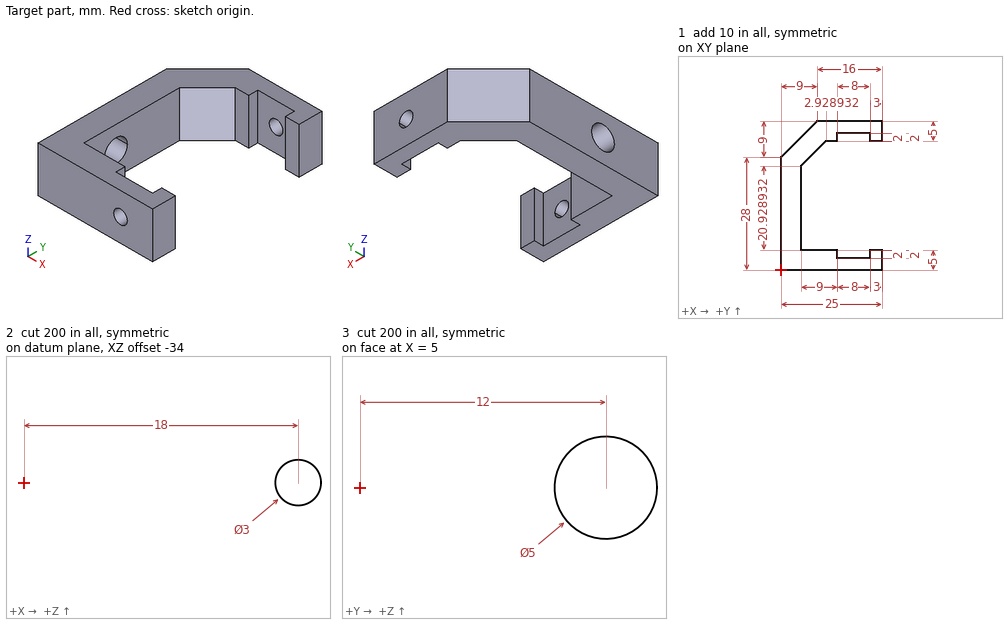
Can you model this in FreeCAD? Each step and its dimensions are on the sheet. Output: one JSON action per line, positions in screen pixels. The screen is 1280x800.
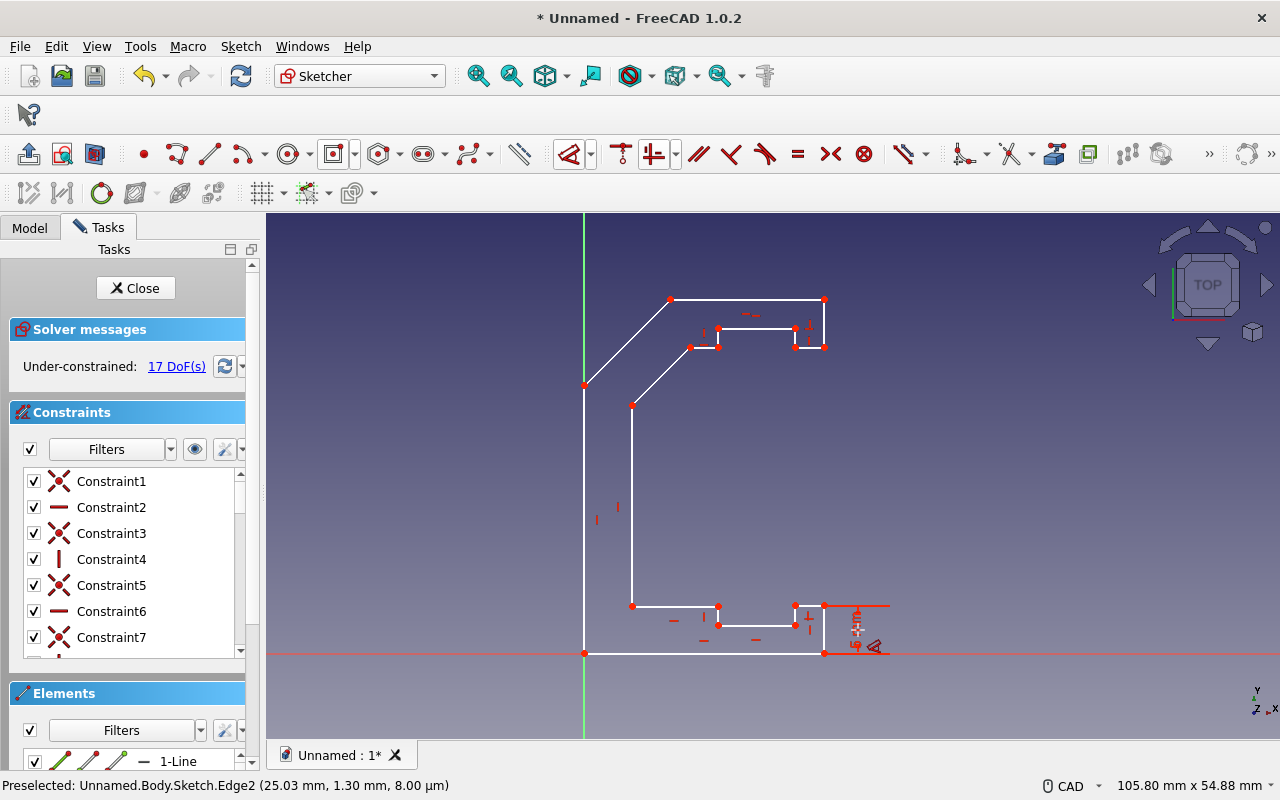
{"action": "scroll", "coordinate": [812, 606], "scroll_direction": "up", "scroll_amount": 2}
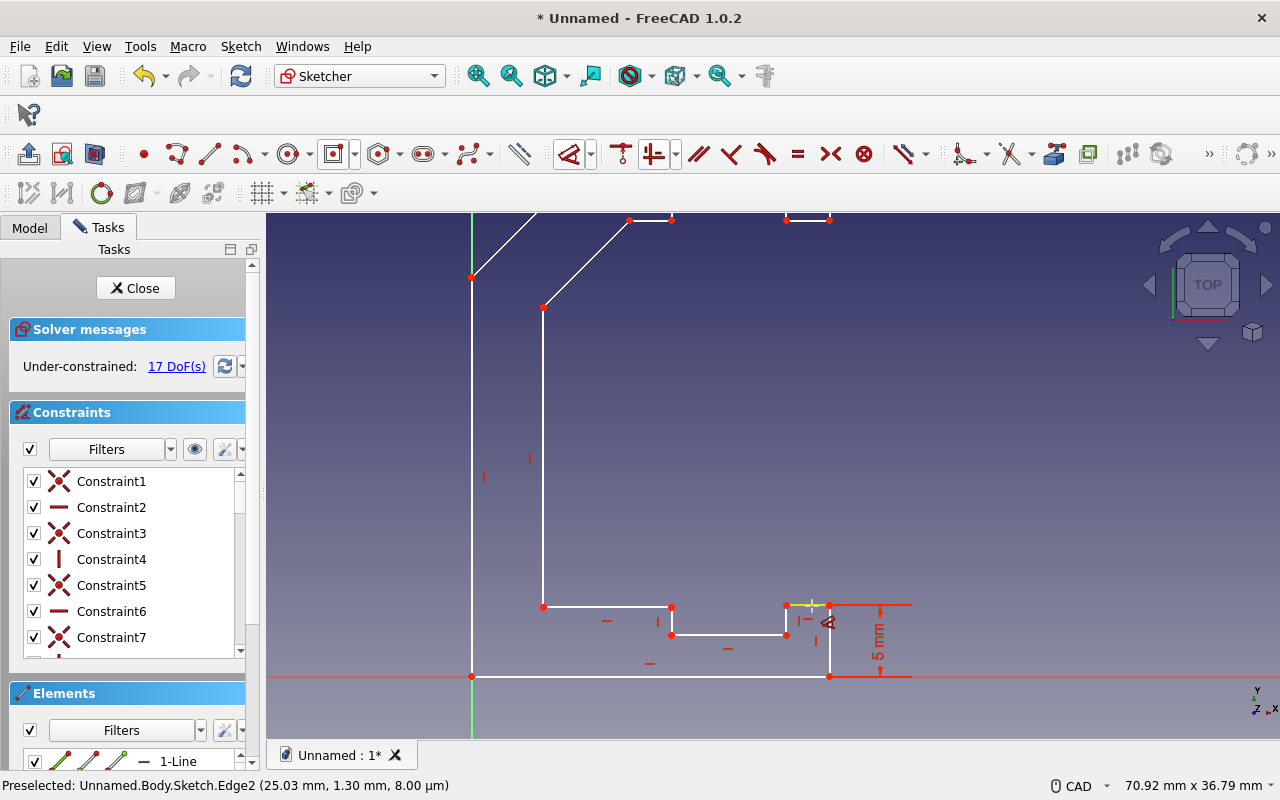
{"action": "left_click", "coordinate": [812, 605]}
{"action": "left_click", "coordinate": [808, 639]}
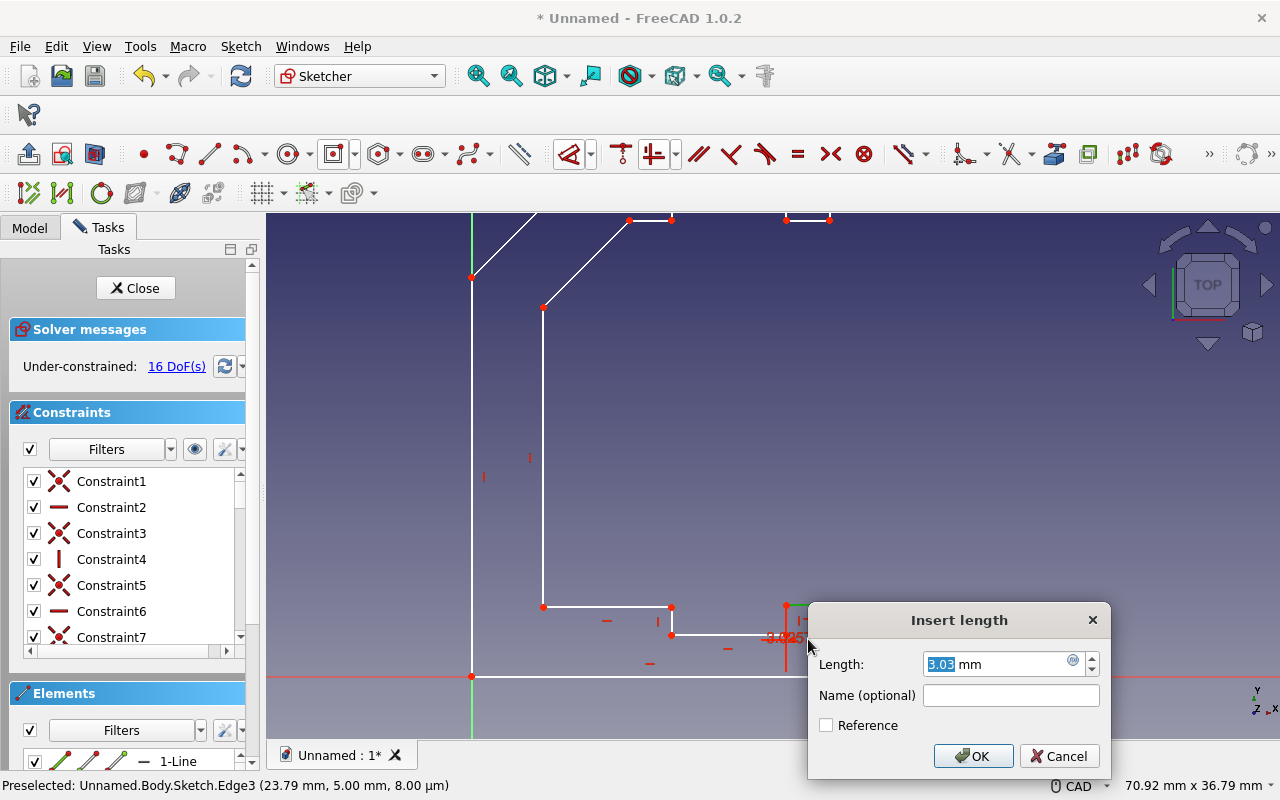
{"action": "type", "text": "3"}
{"action": "key", "text": "Return"}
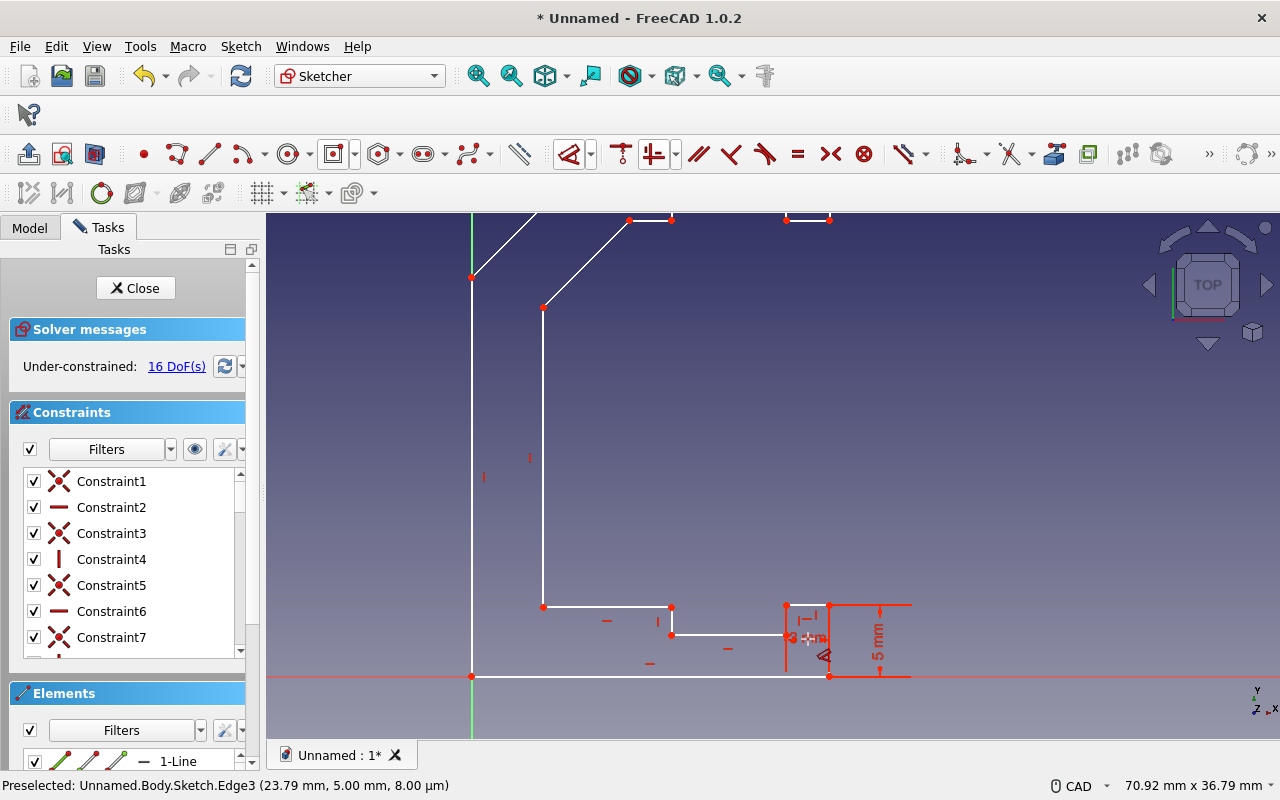
{"action": "scroll", "coordinate": [786, 614], "scroll_direction": "up", "scroll_amount": 3}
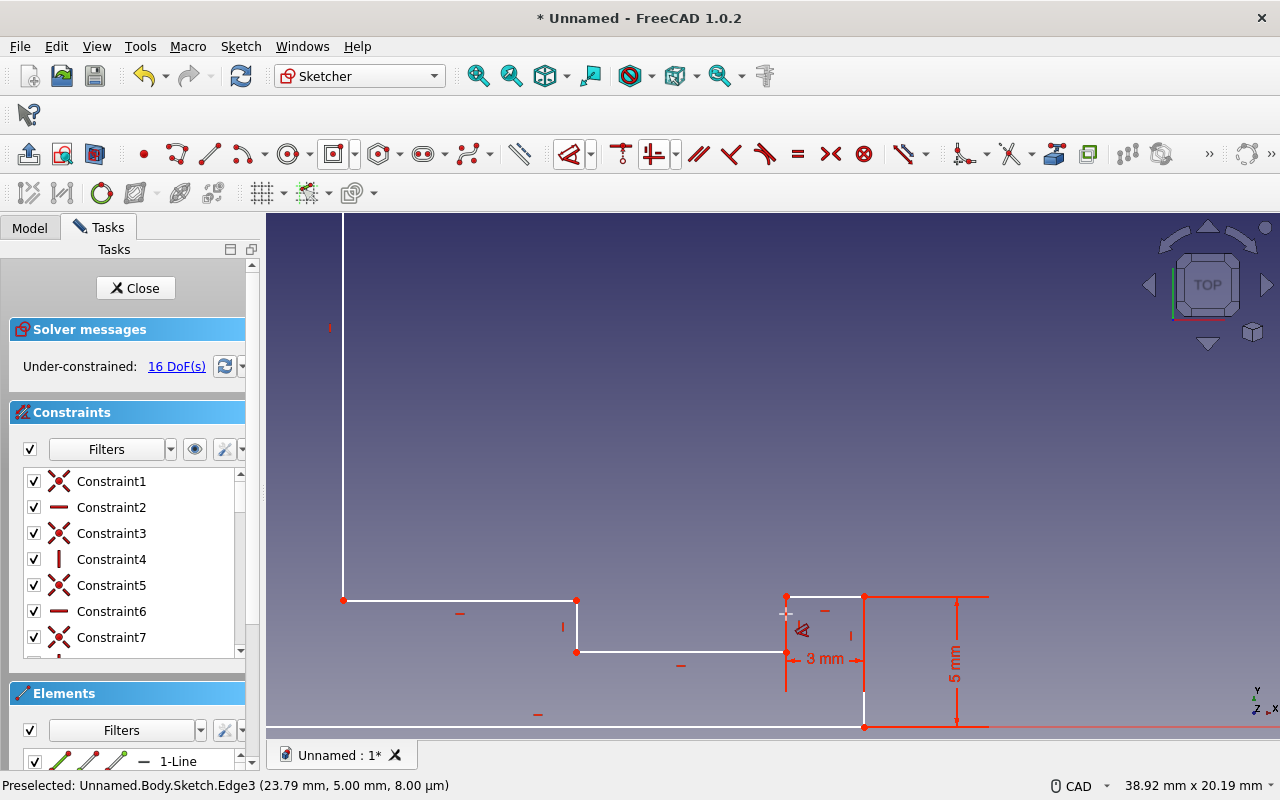
{"action": "left_click", "coordinate": [786, 614]}
{"action": "left_click", "coordinate": [820, 625]}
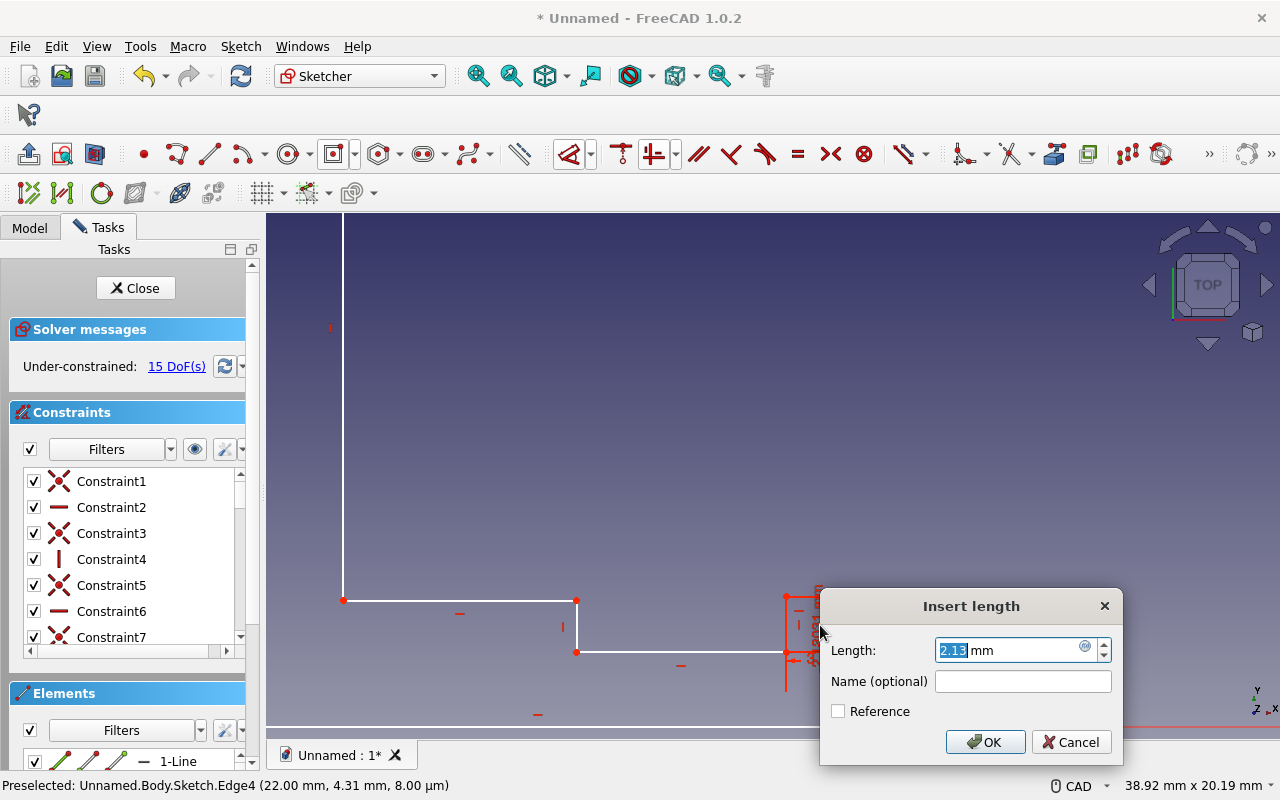
{"action": "type", "text": "2"}
{"action": "key", "text": "Return"}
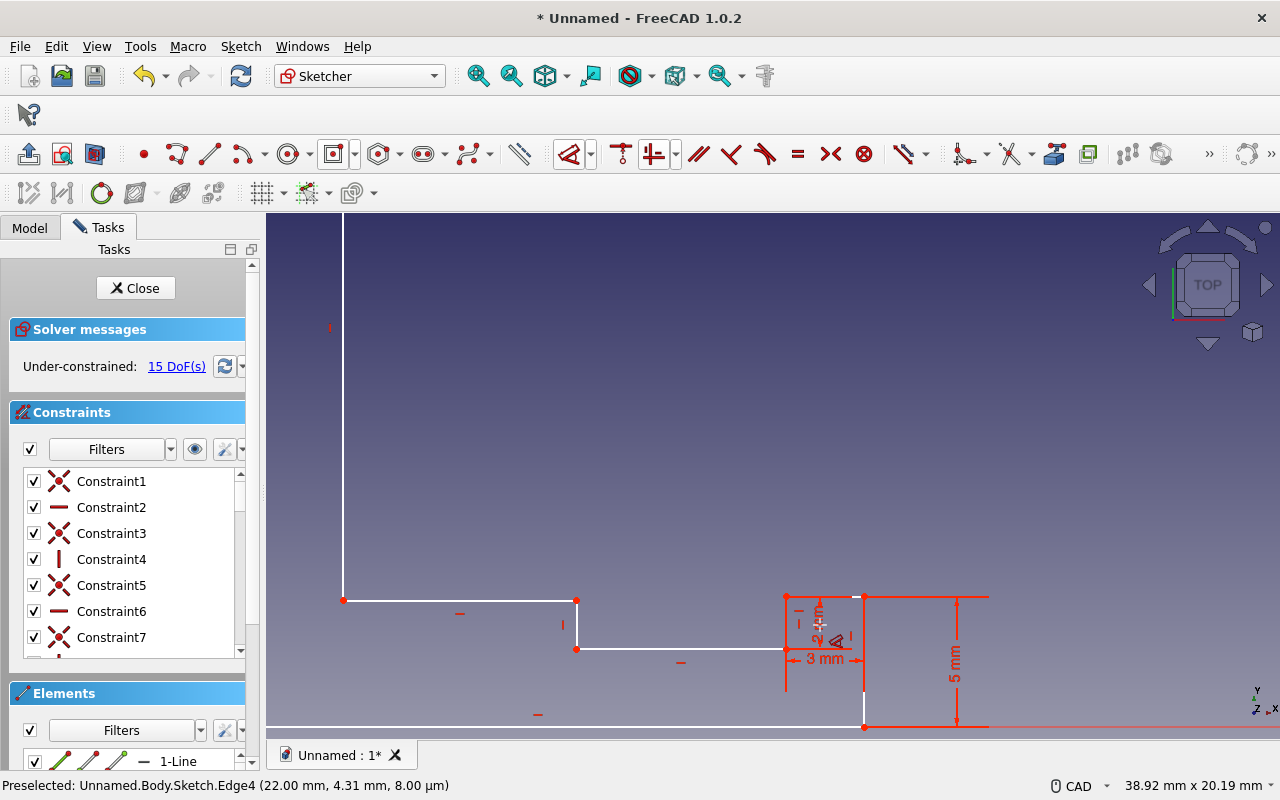
{"action": "left_click", "coordinate": [723, 649]}
{"action": "left_click", "coordinate": [682, 683]}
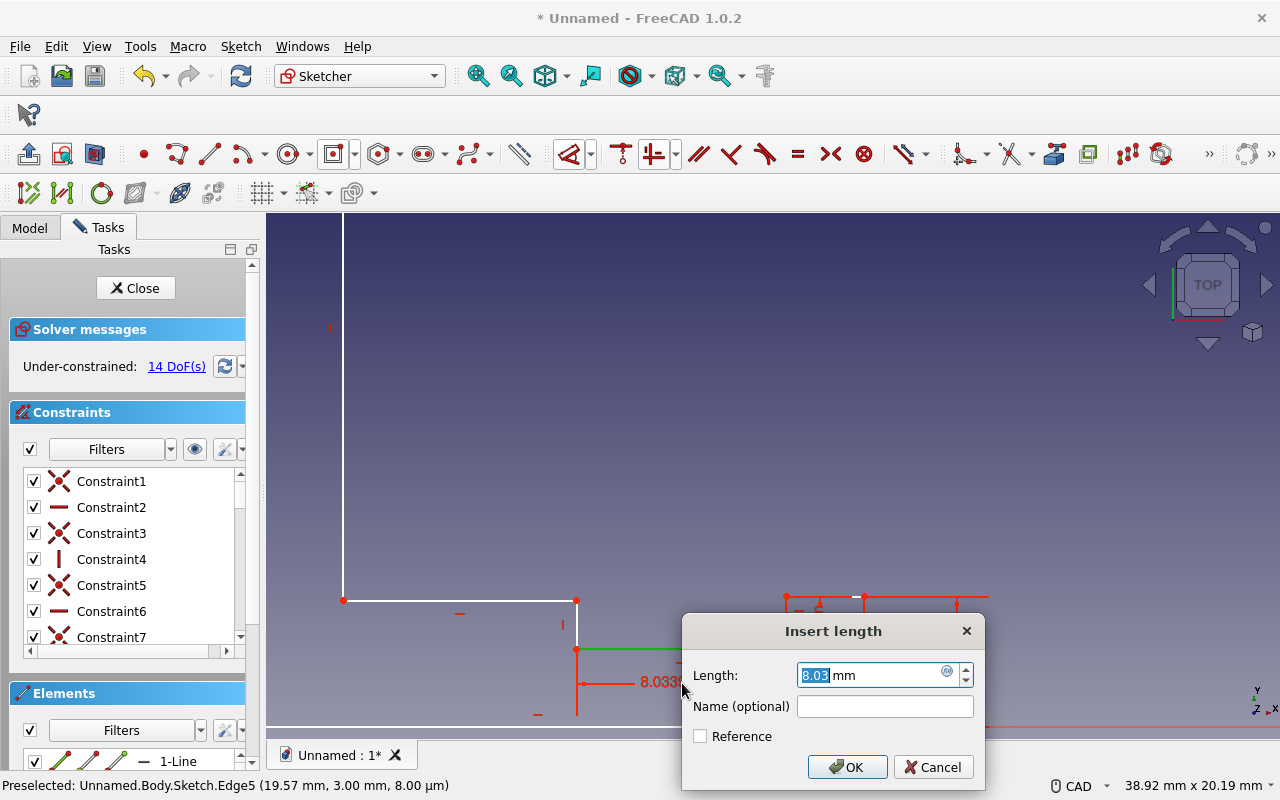
{"action": "type", "text": "8"}
{"action": "key", "text": "Return"}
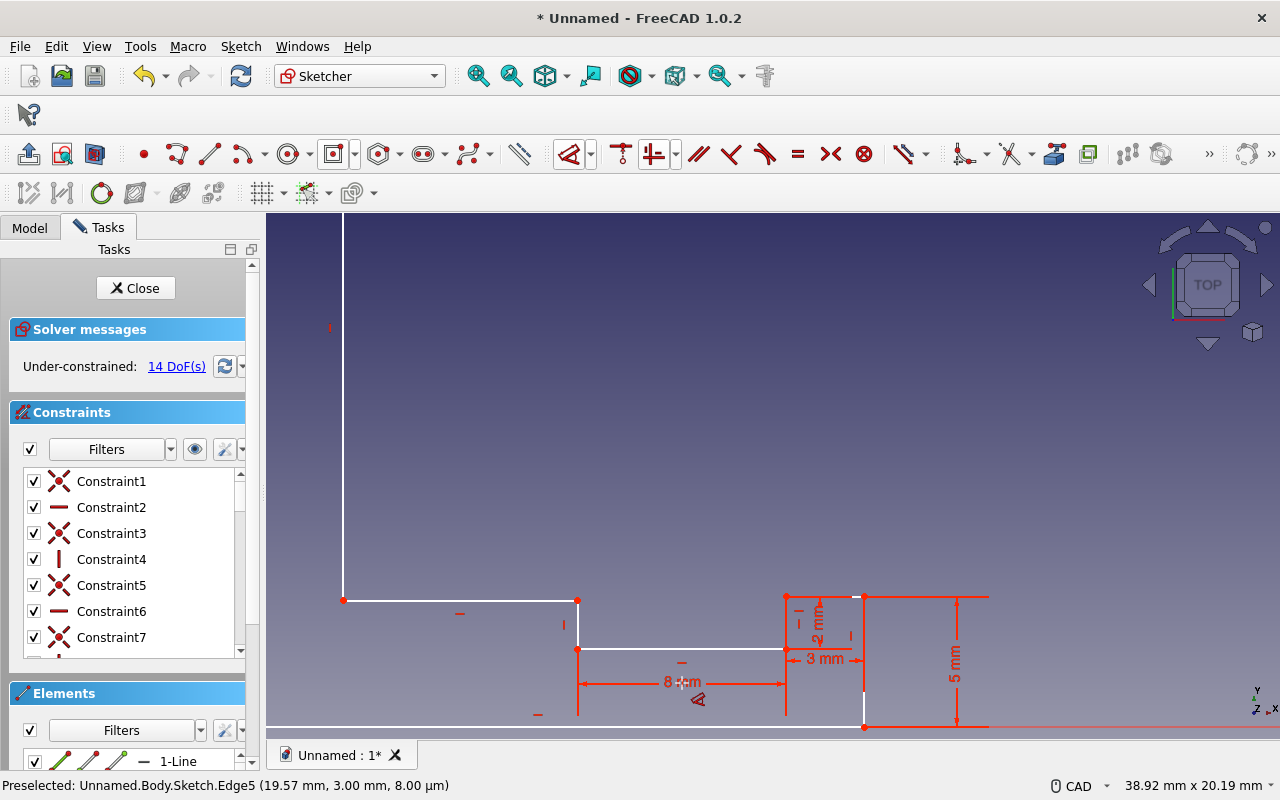
{"action": "left_click", "coordinate": [578, 635]}
{"action": "left_click", "coordinate": [612, 625]}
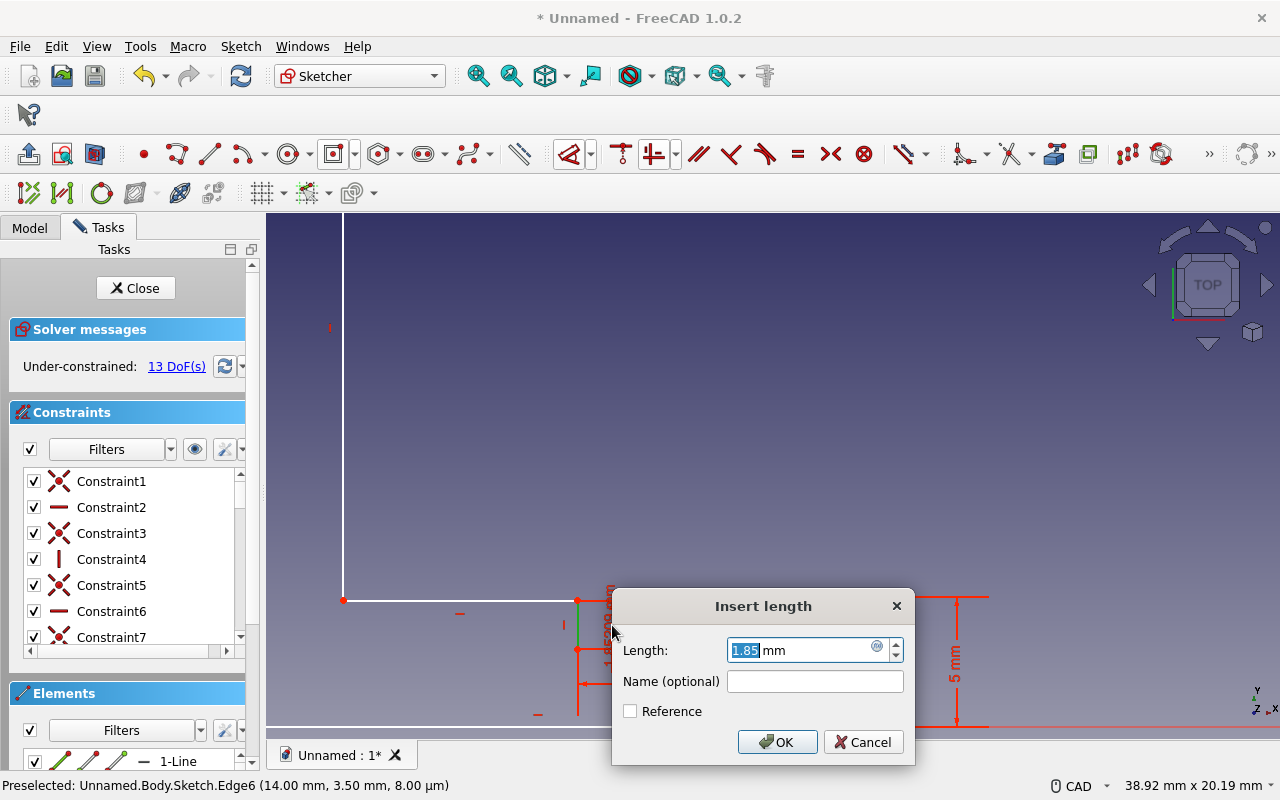
{"action": "type", "text": "2"}
{"action": "key", "text": "Return"}